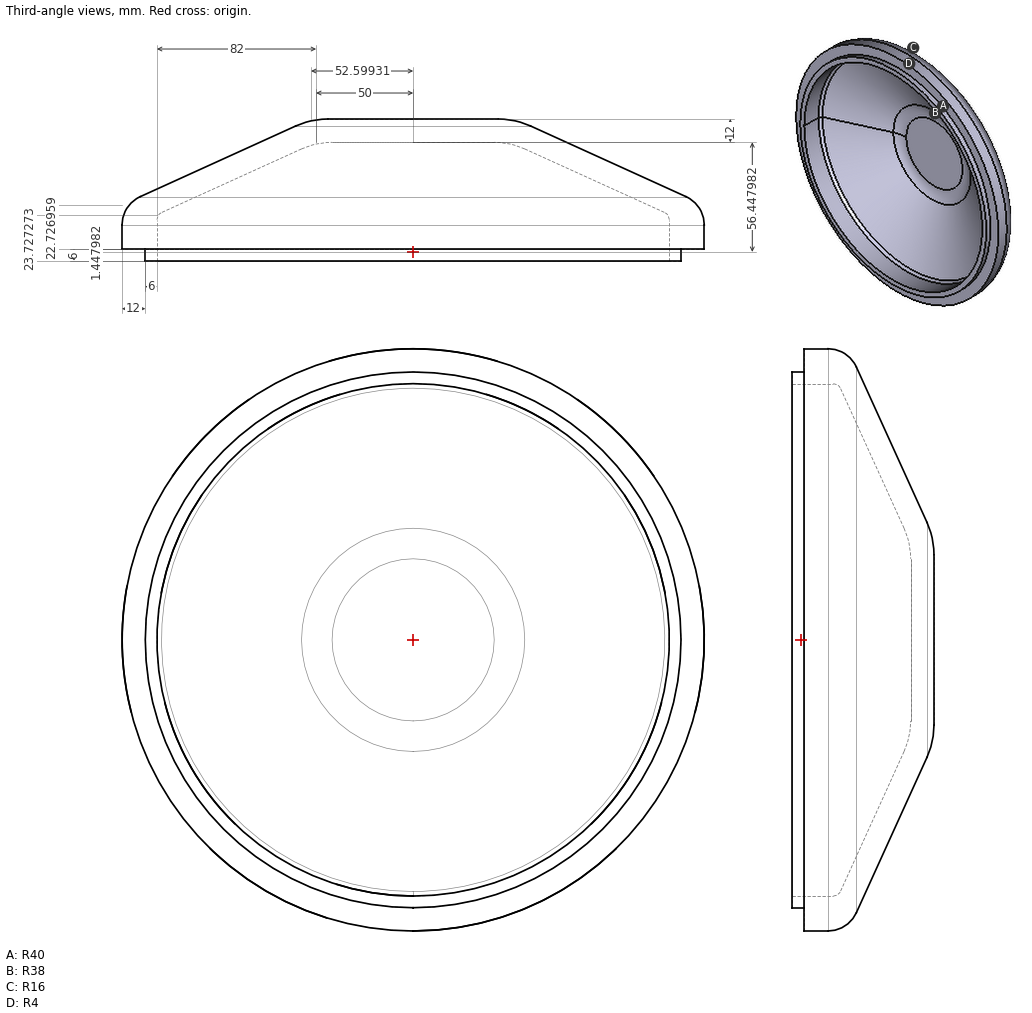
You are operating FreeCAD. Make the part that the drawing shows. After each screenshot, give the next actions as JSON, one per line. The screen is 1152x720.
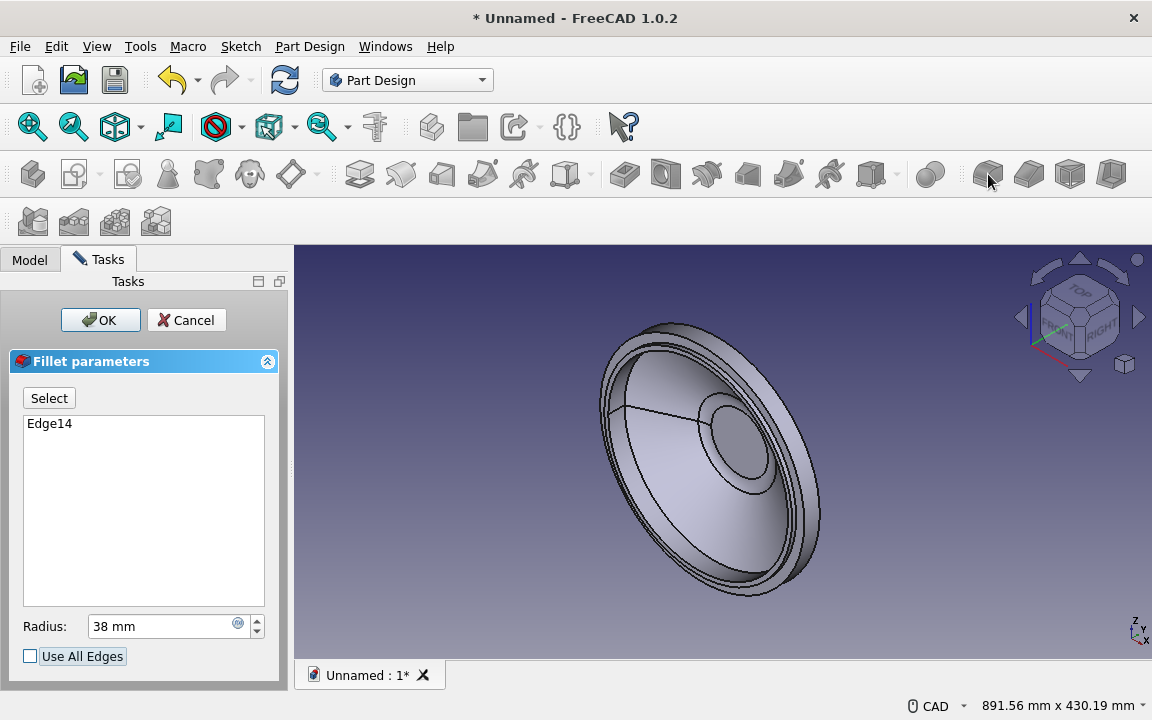
{"action": "left_click", "coordinate": [101, 320]}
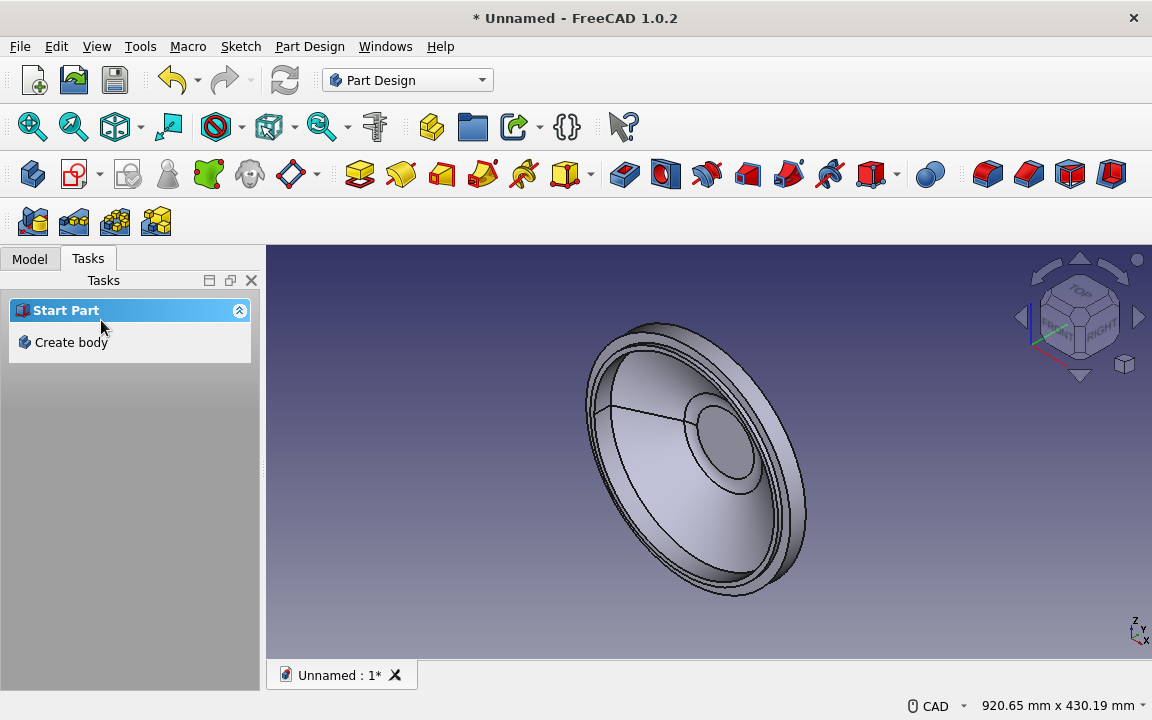
{"action": "key", "text": "2"}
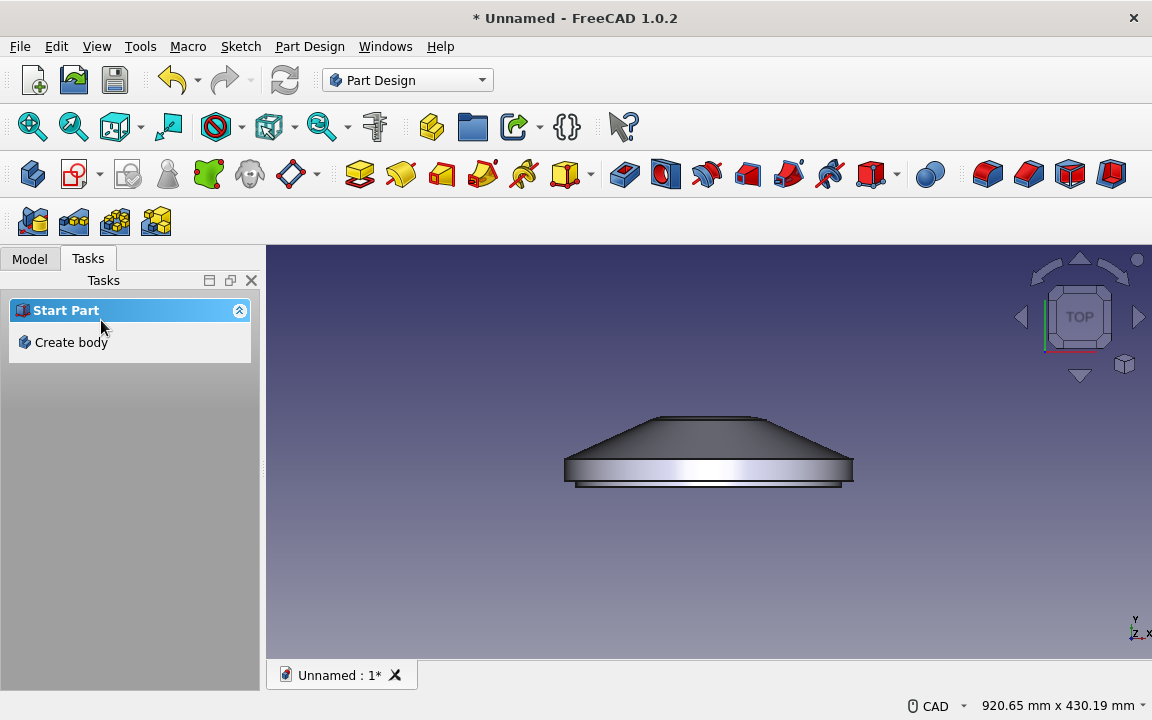
{"action": "left_click", "coordinate": [33, 128]}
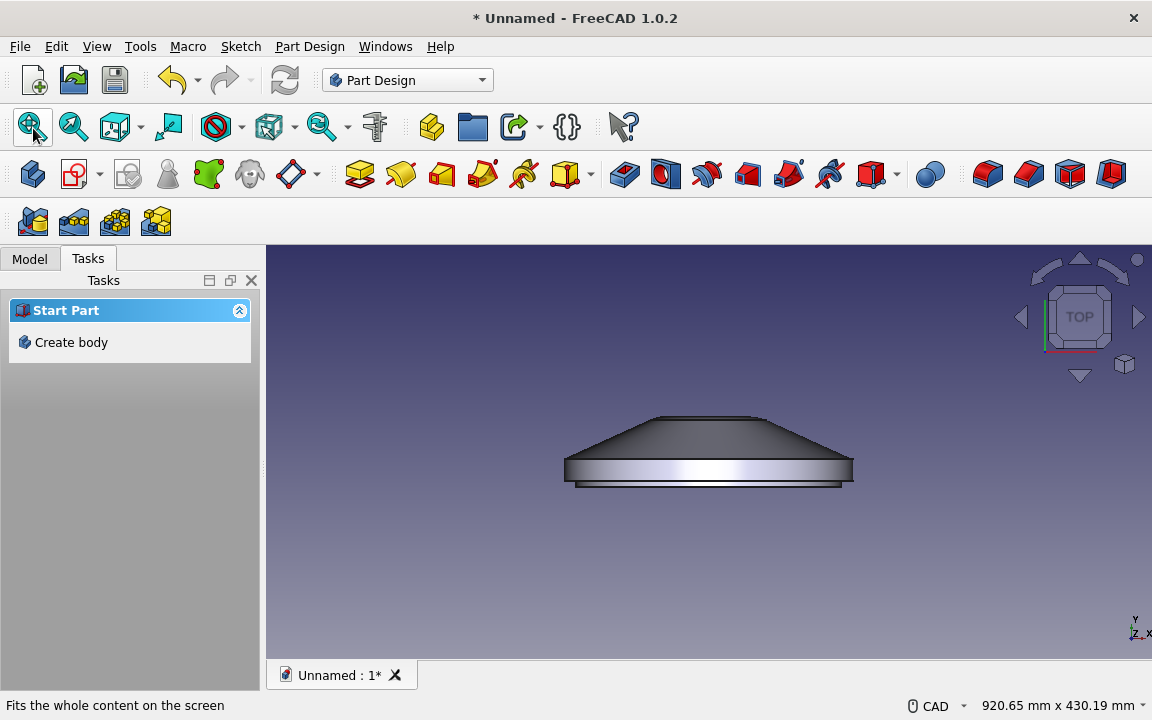
{"action": "left_click", "coordinate": [826, 458]}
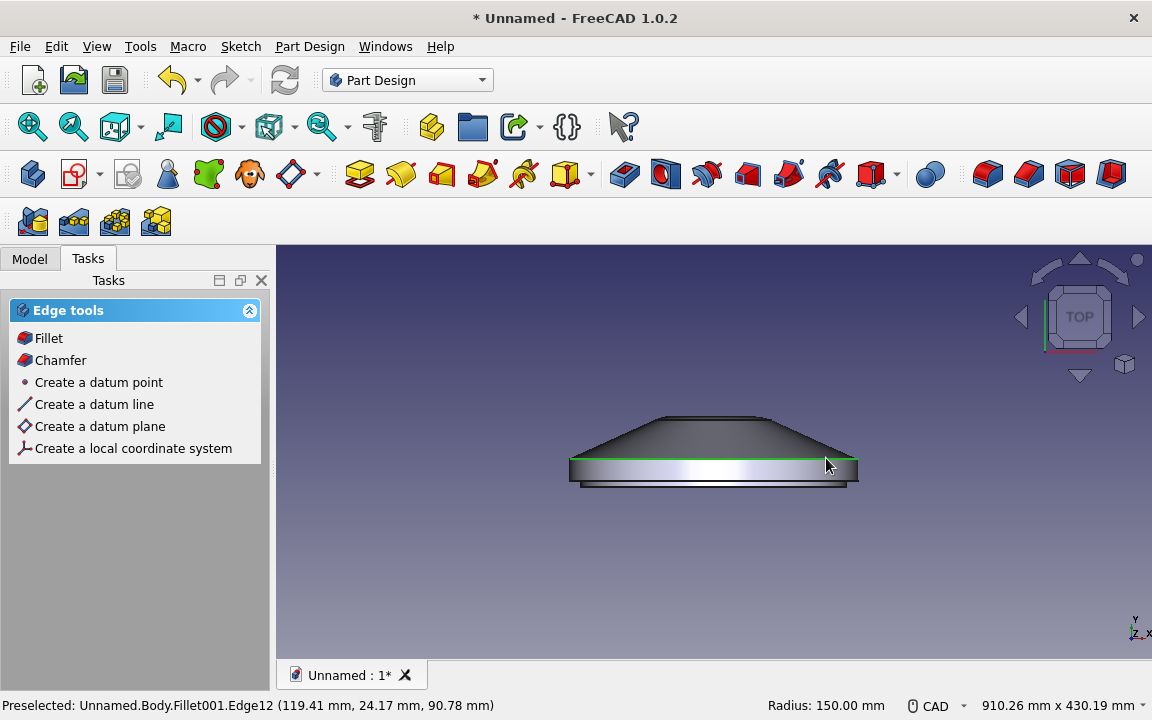
{"action": "left_click", "coordinate": [988, 174]}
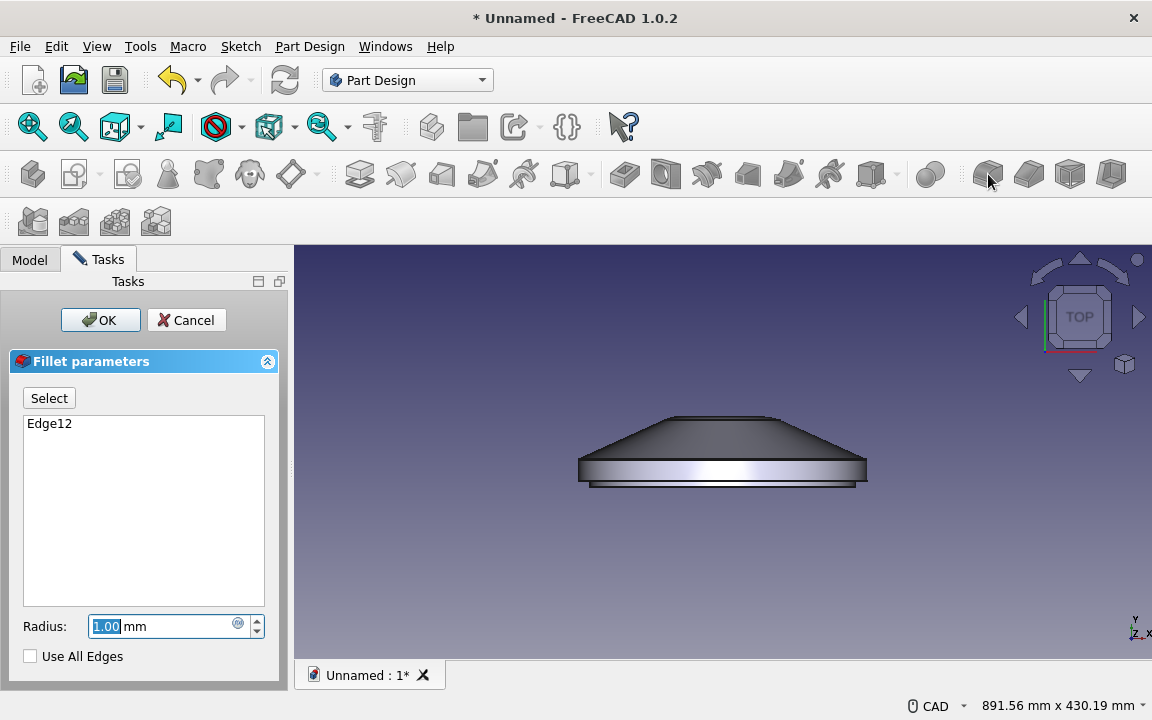
{"action": "type", "text": "16"}
{"action": "key", "text": "Tab"}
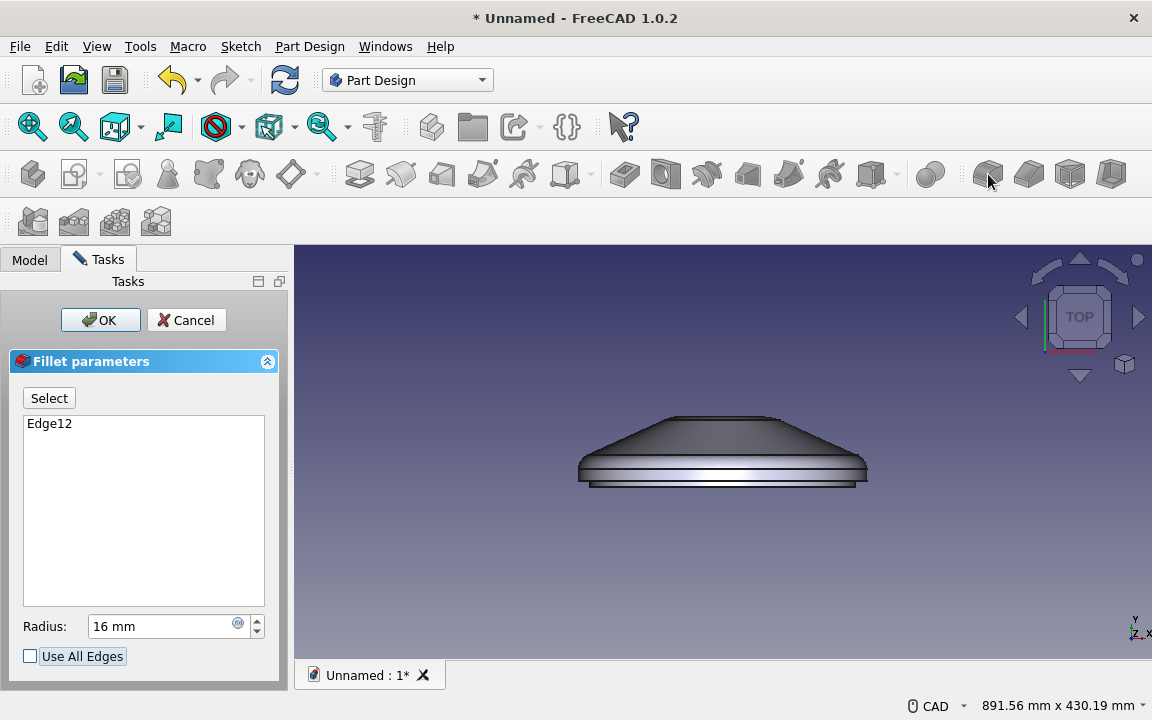
{"action": "left_click", "coordinate": [101, 320]}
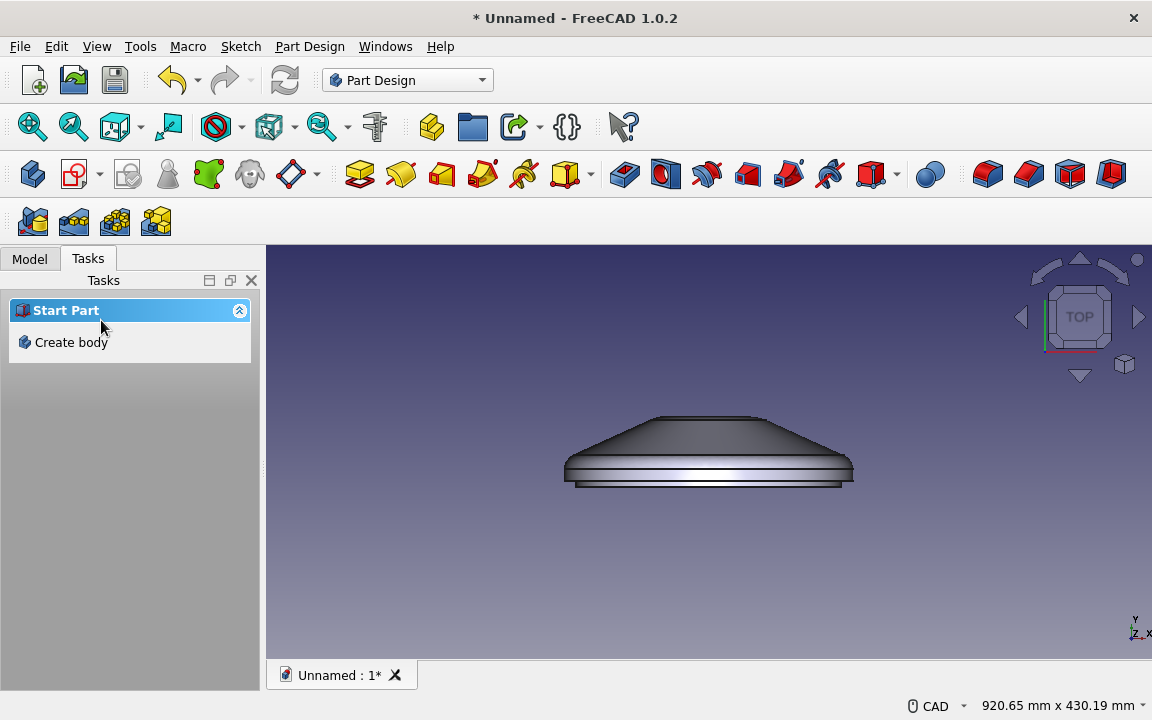
{"action": "key", "text": "v f"}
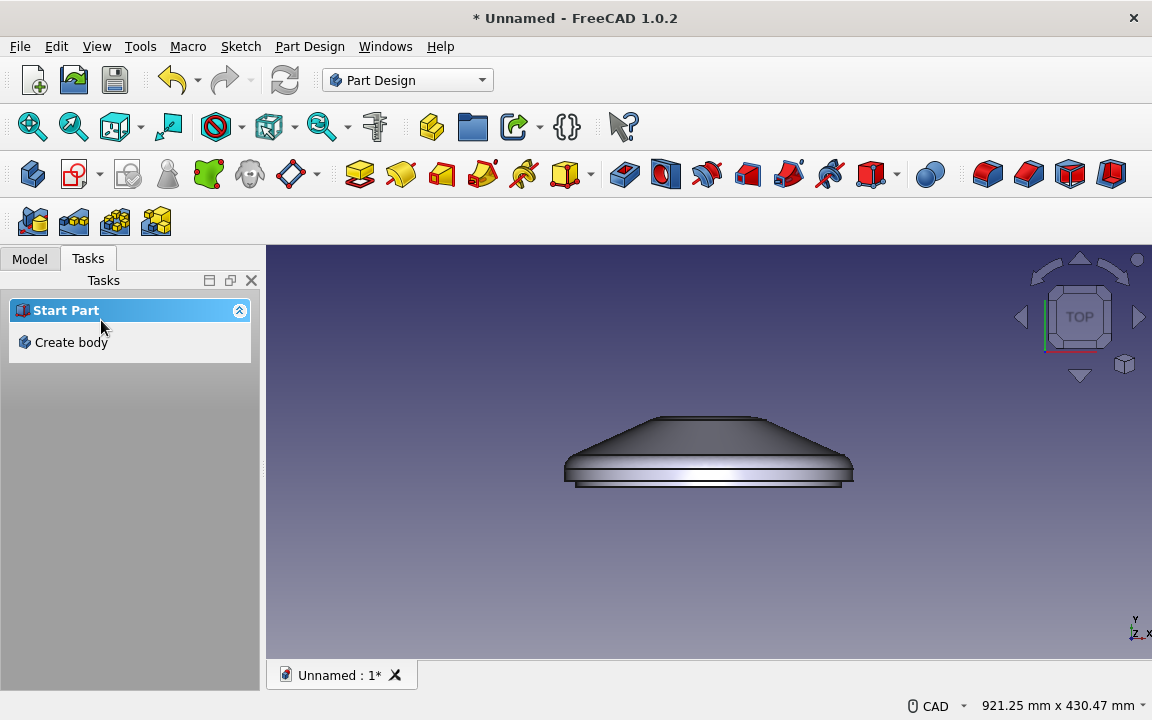
{"action": "key", "text": "0"}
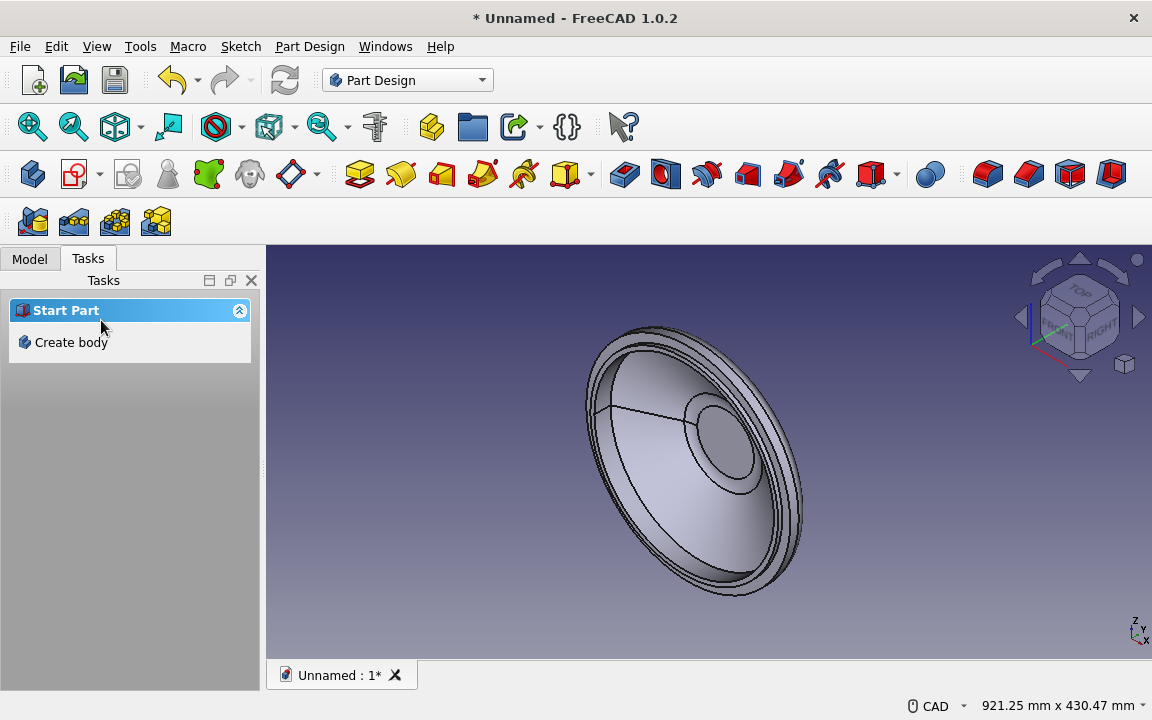
{"action": "key", "text": "2"}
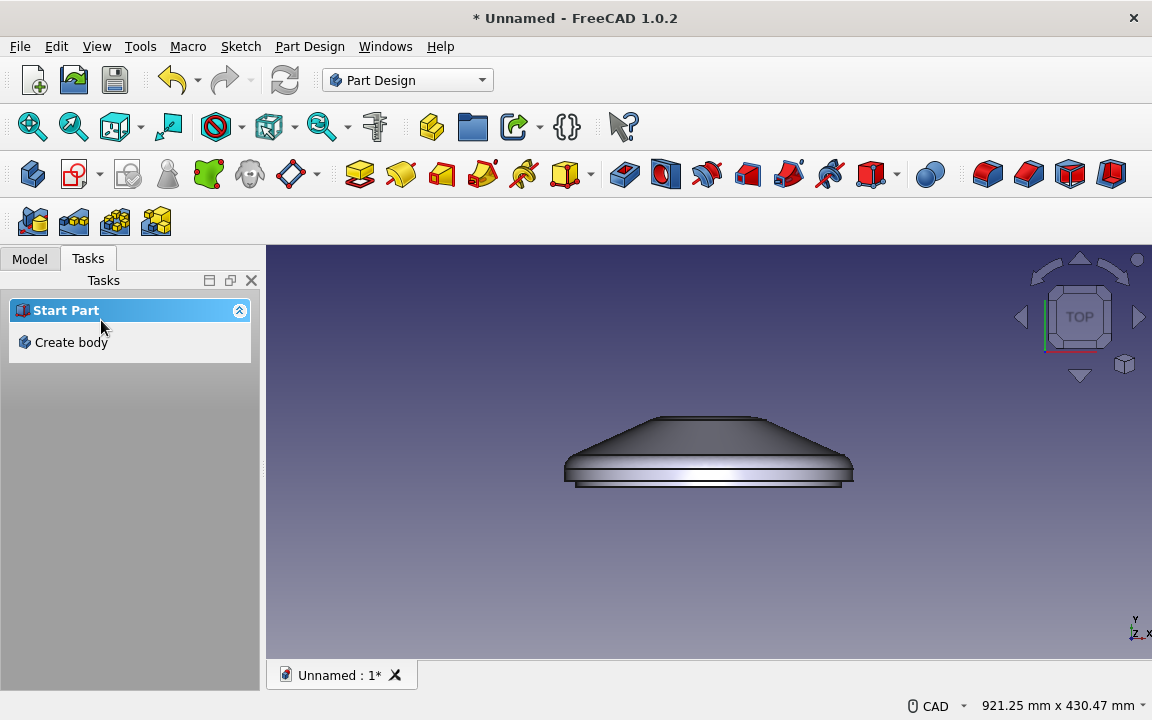
{"action": "left_click", "coordinate": [33, 128]}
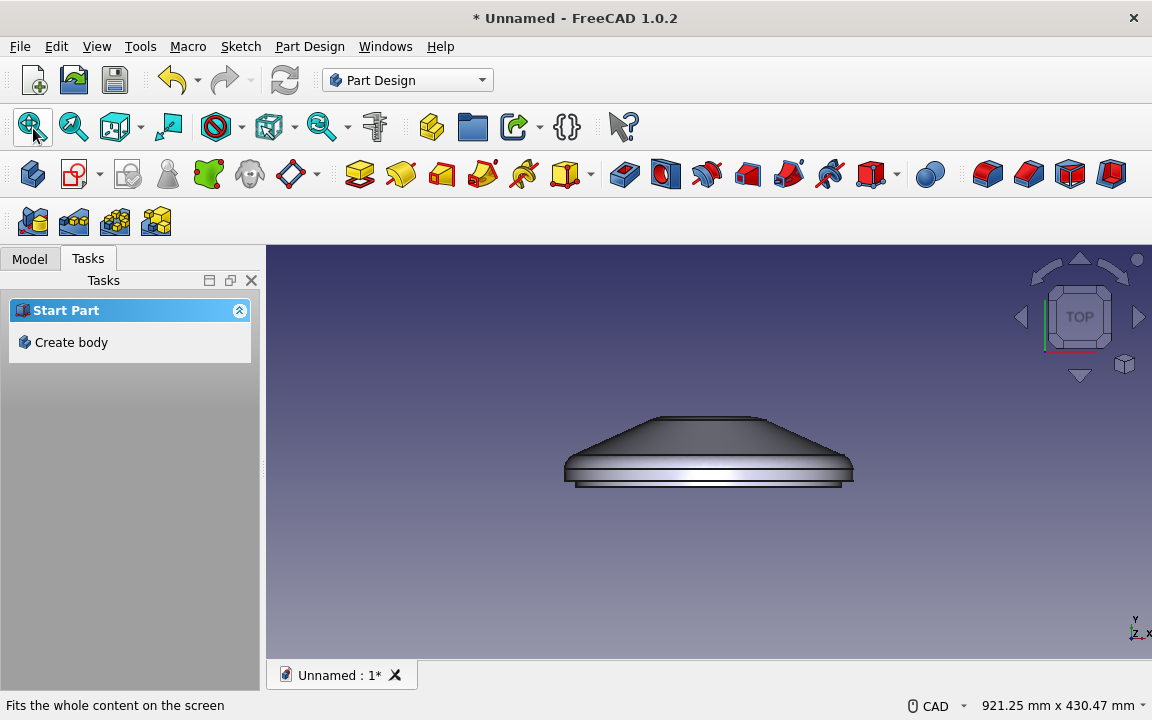
{"action": "key", "text": "1"}